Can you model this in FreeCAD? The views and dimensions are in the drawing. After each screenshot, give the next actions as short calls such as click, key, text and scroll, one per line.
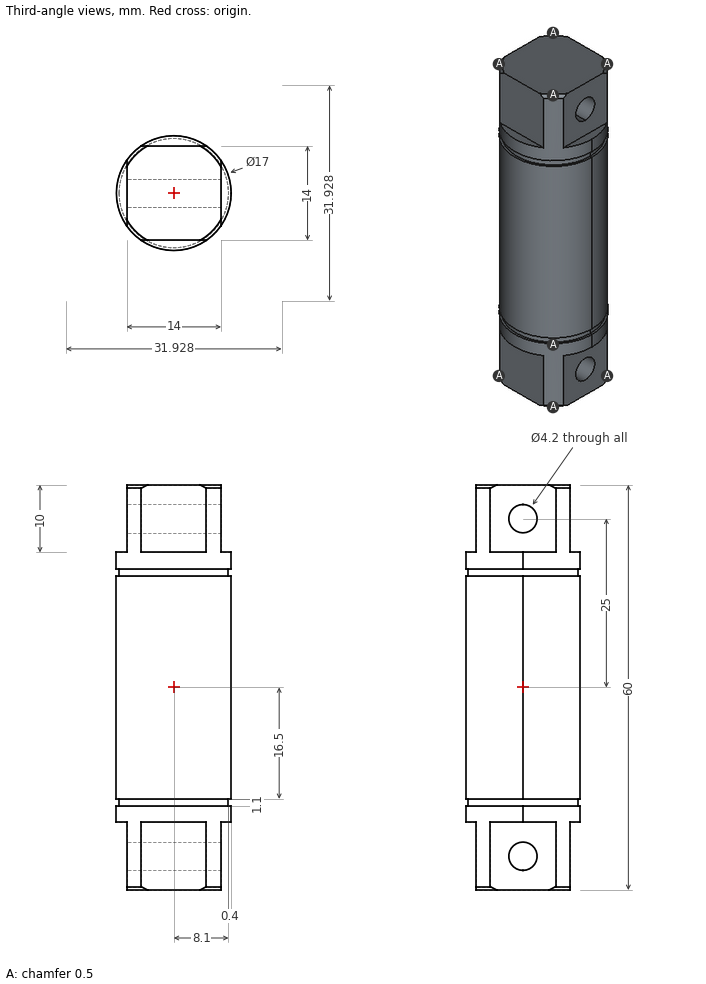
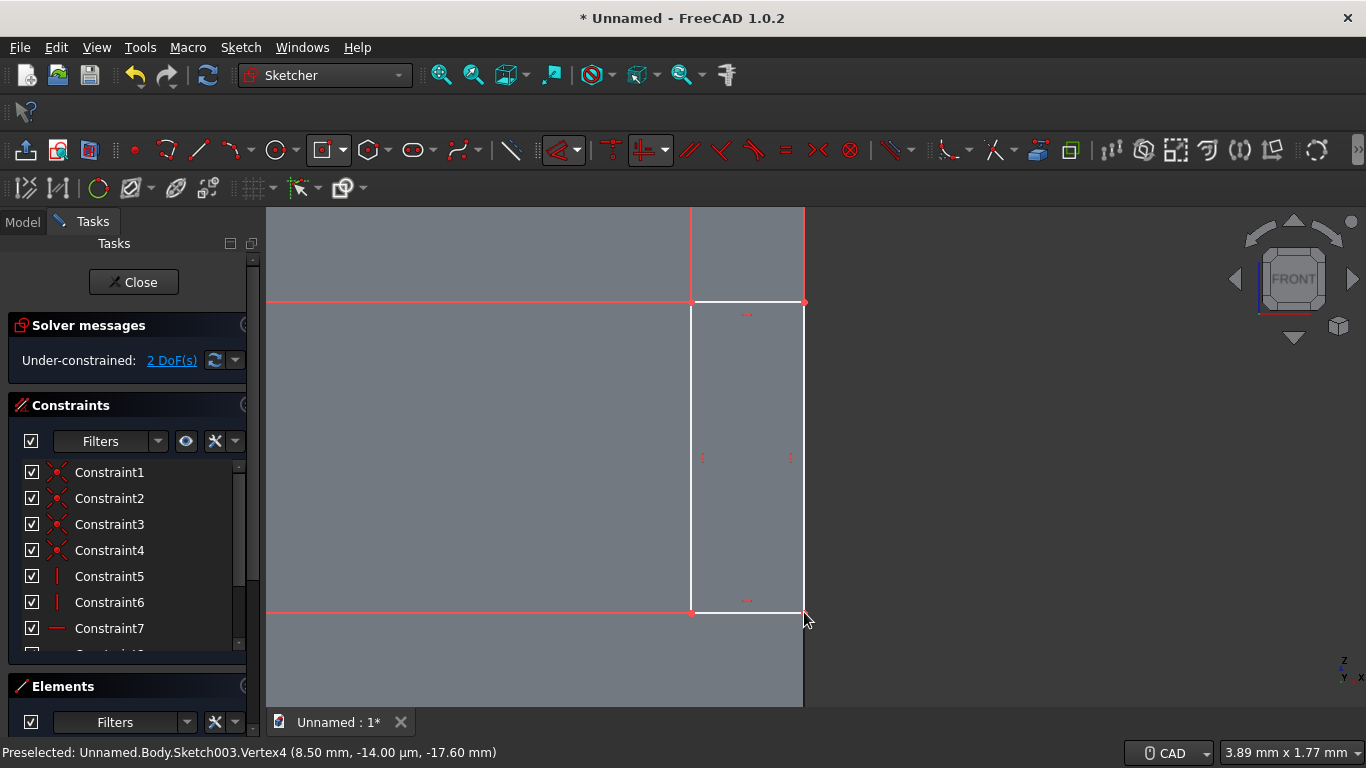
click(691, 302)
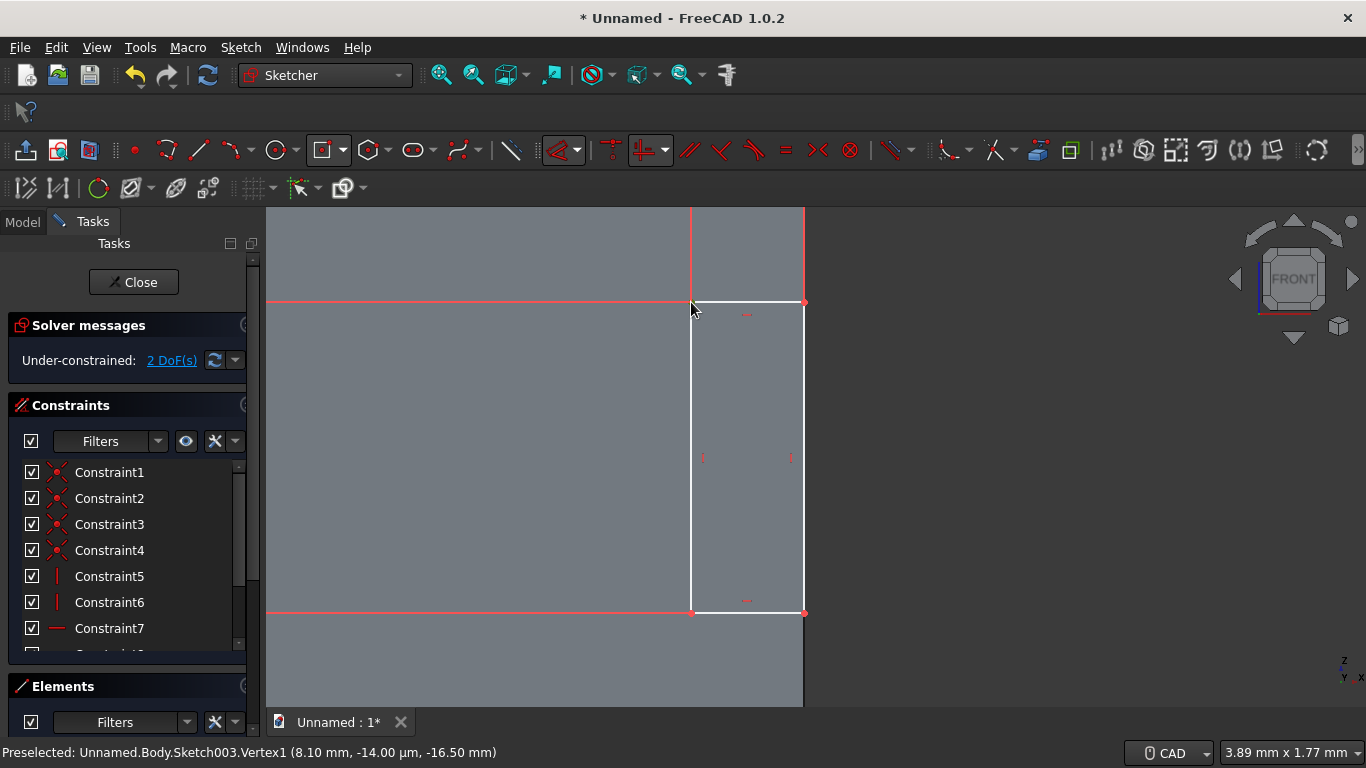
key(l)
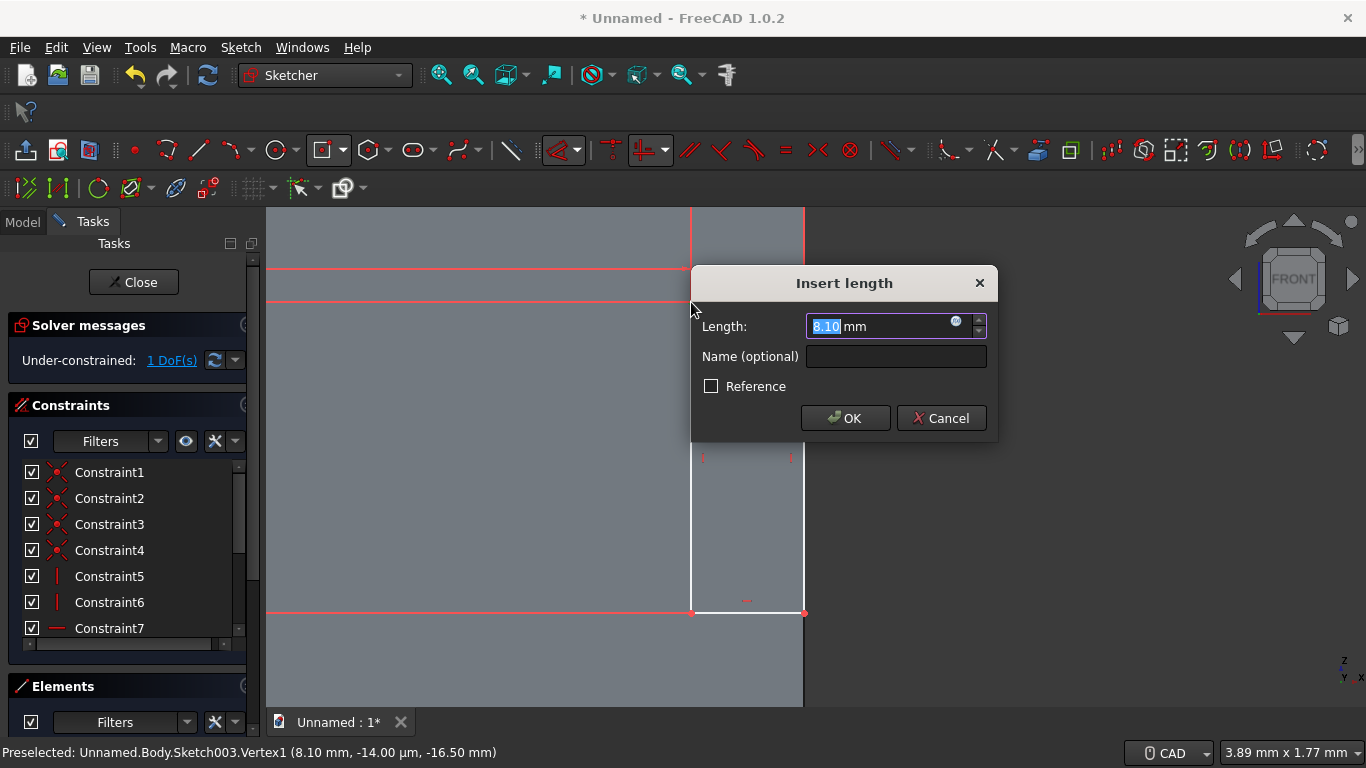
text(8.1)
key(Return)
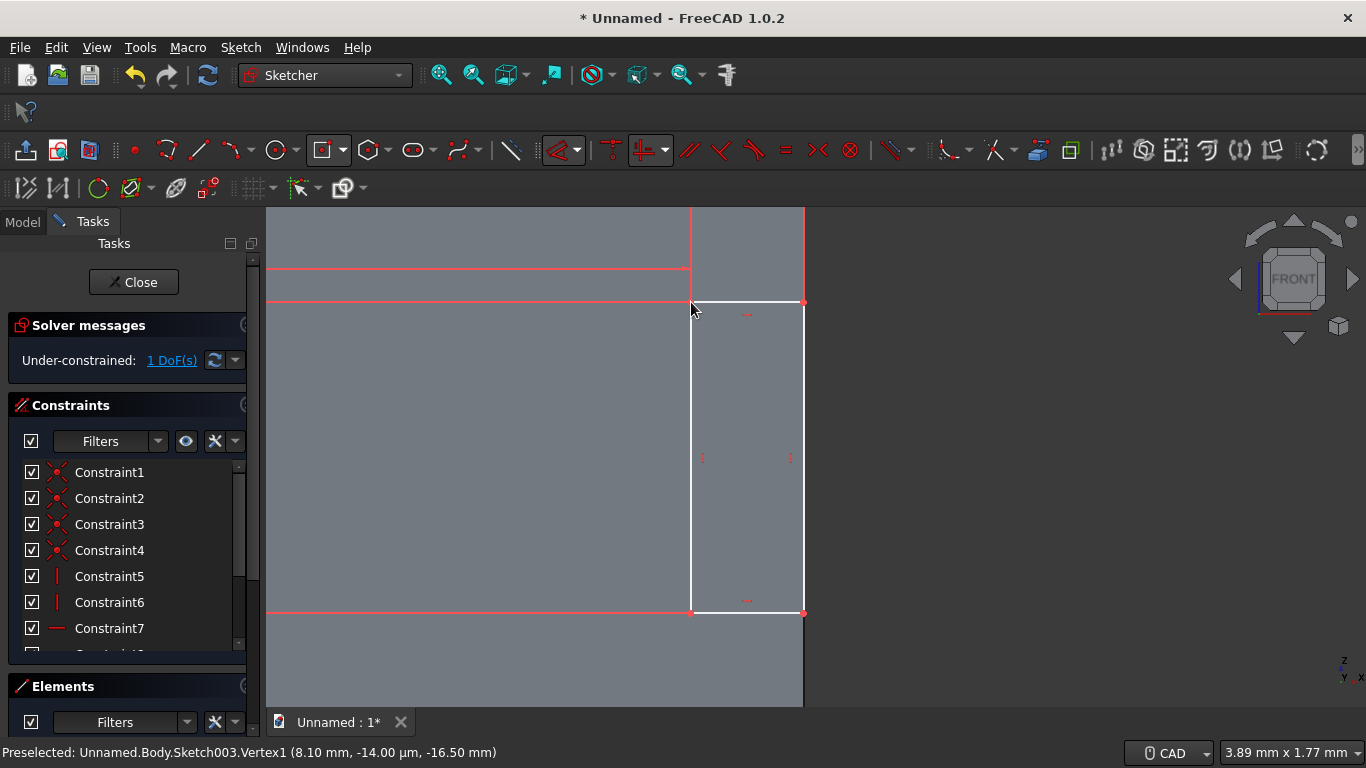
click(691, 302)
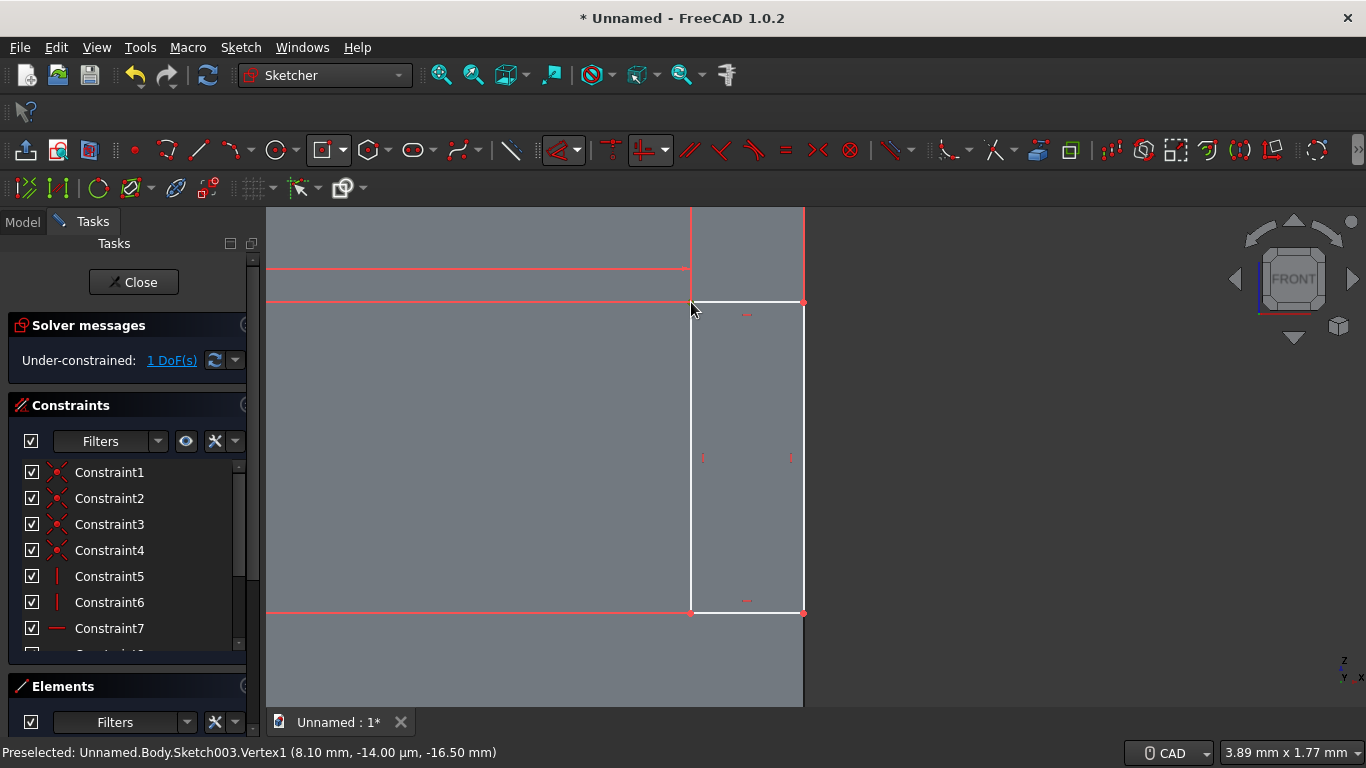
key(i)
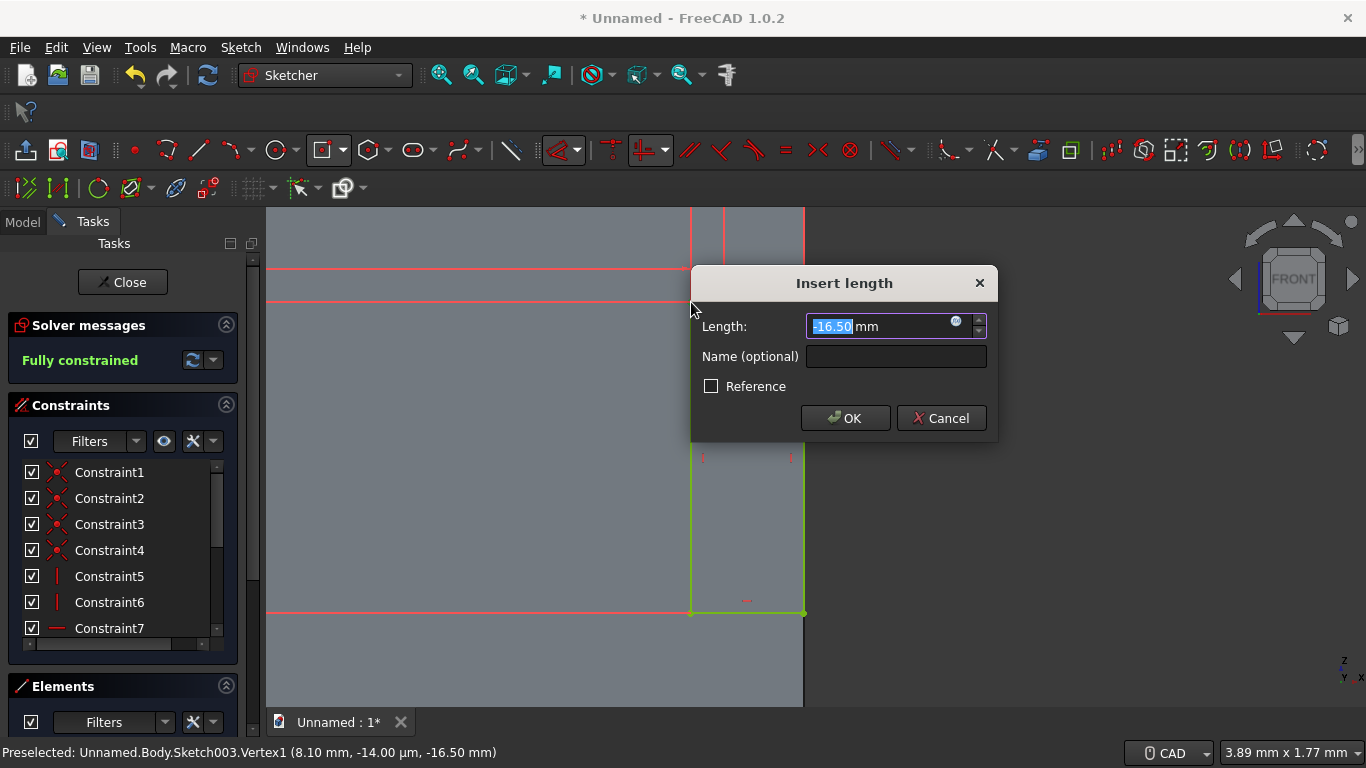
text(-16.5)
key(Return)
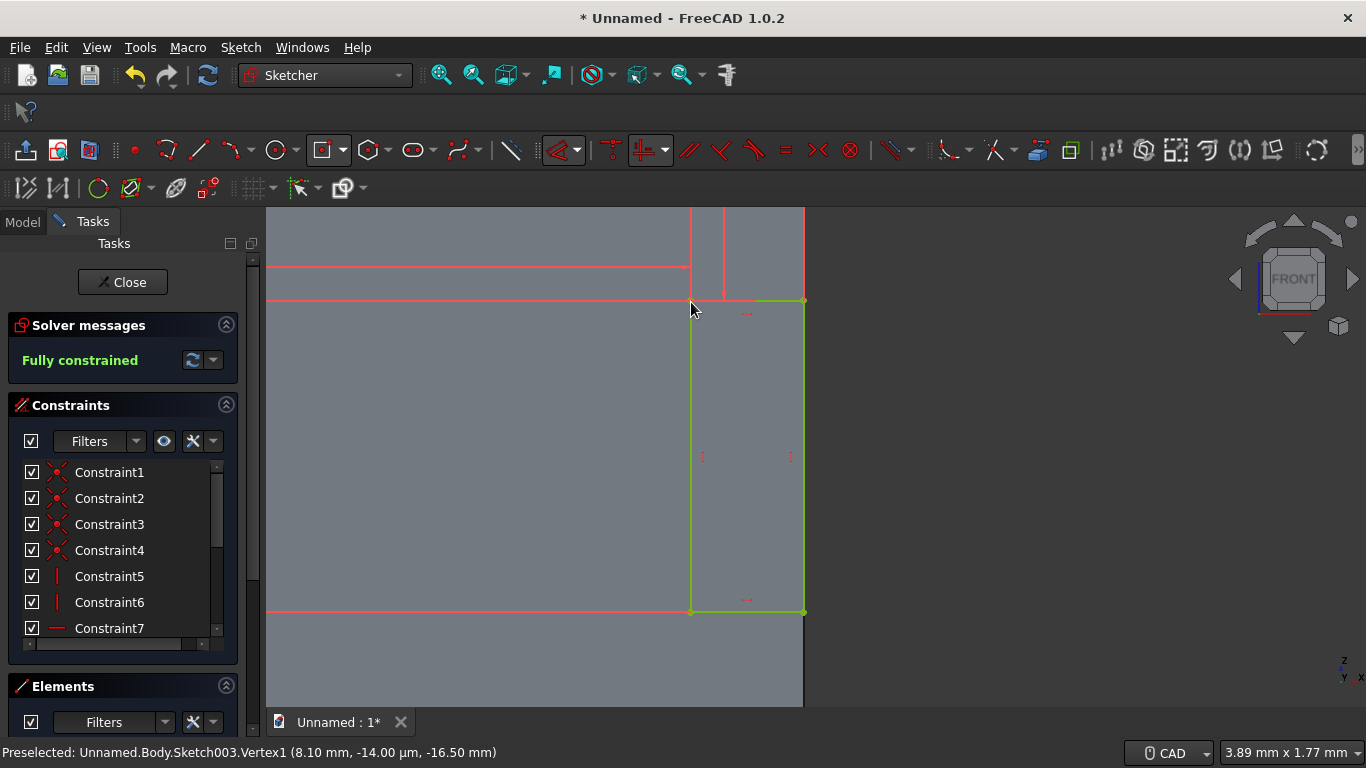
click(123, 282)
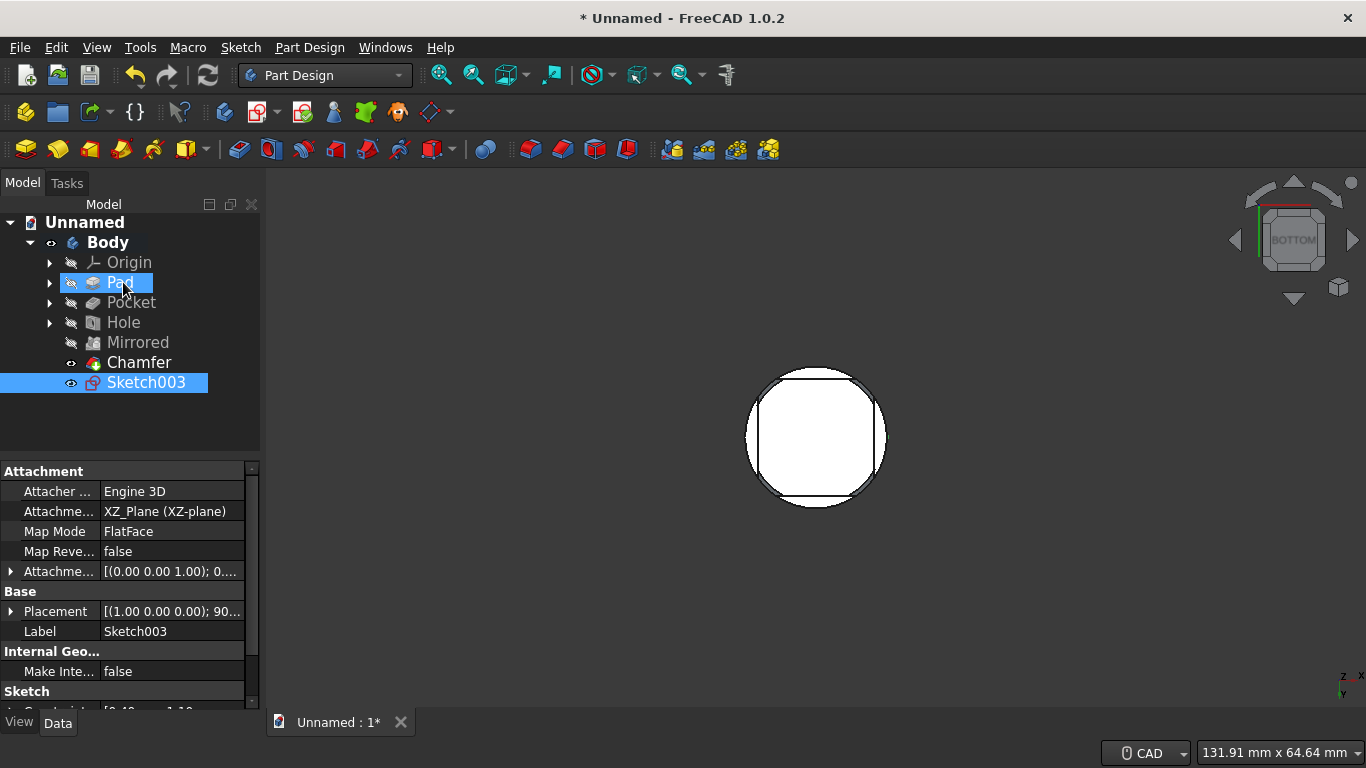
click(304, 150)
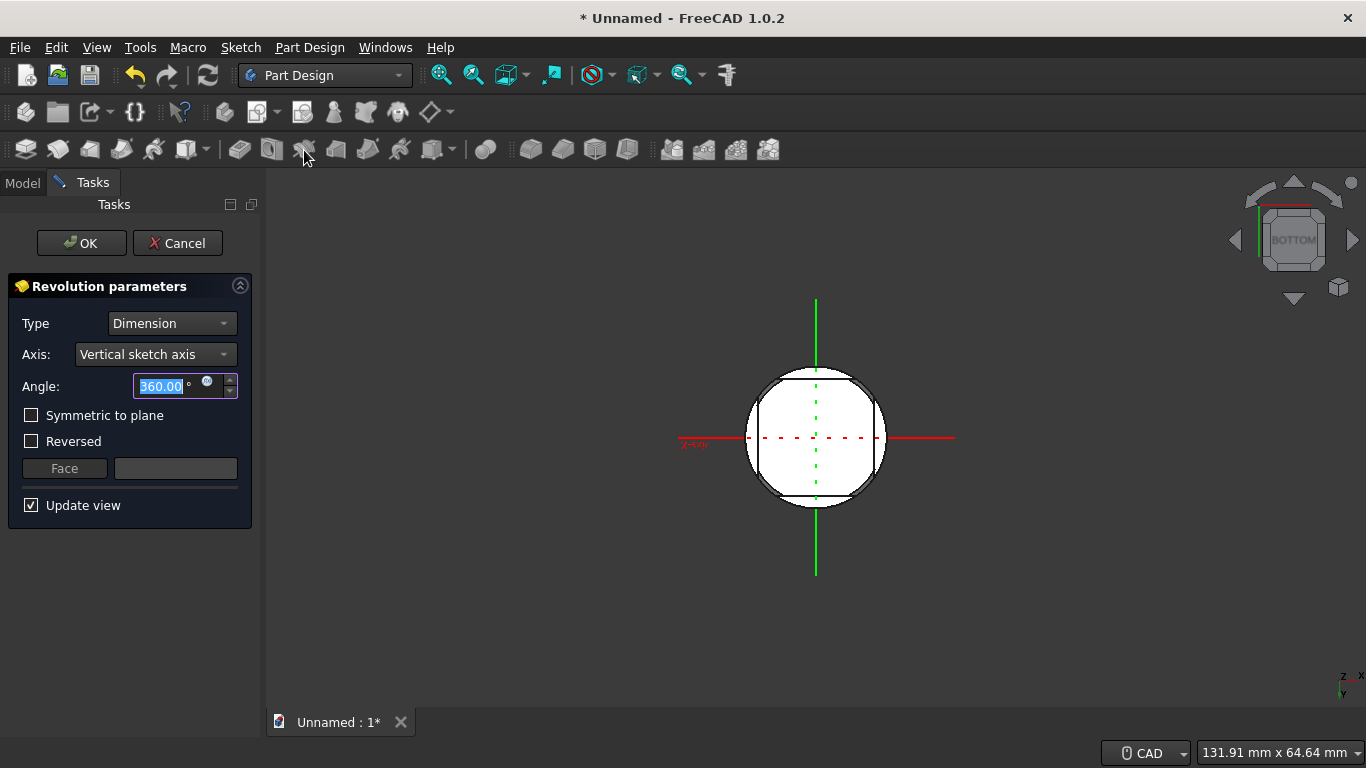
click(82, 243)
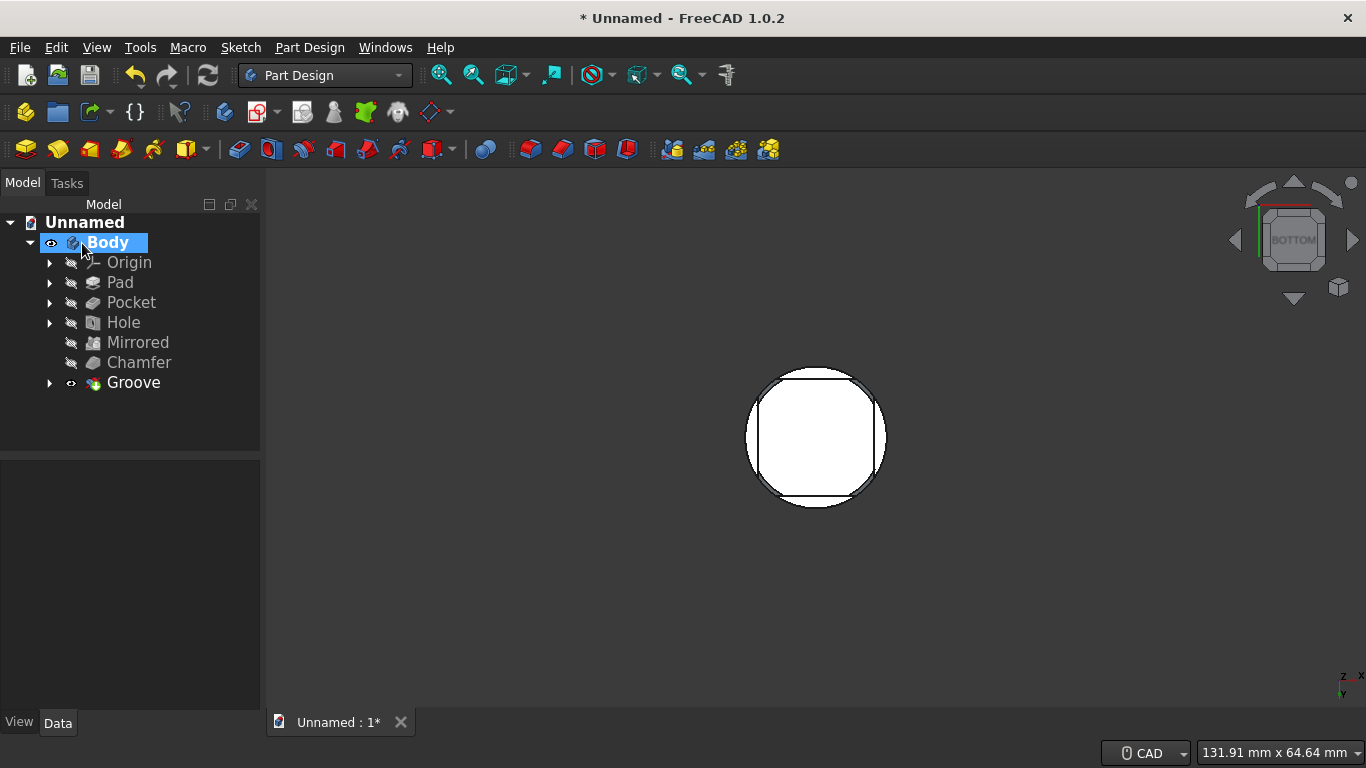
key(v)
key(f)